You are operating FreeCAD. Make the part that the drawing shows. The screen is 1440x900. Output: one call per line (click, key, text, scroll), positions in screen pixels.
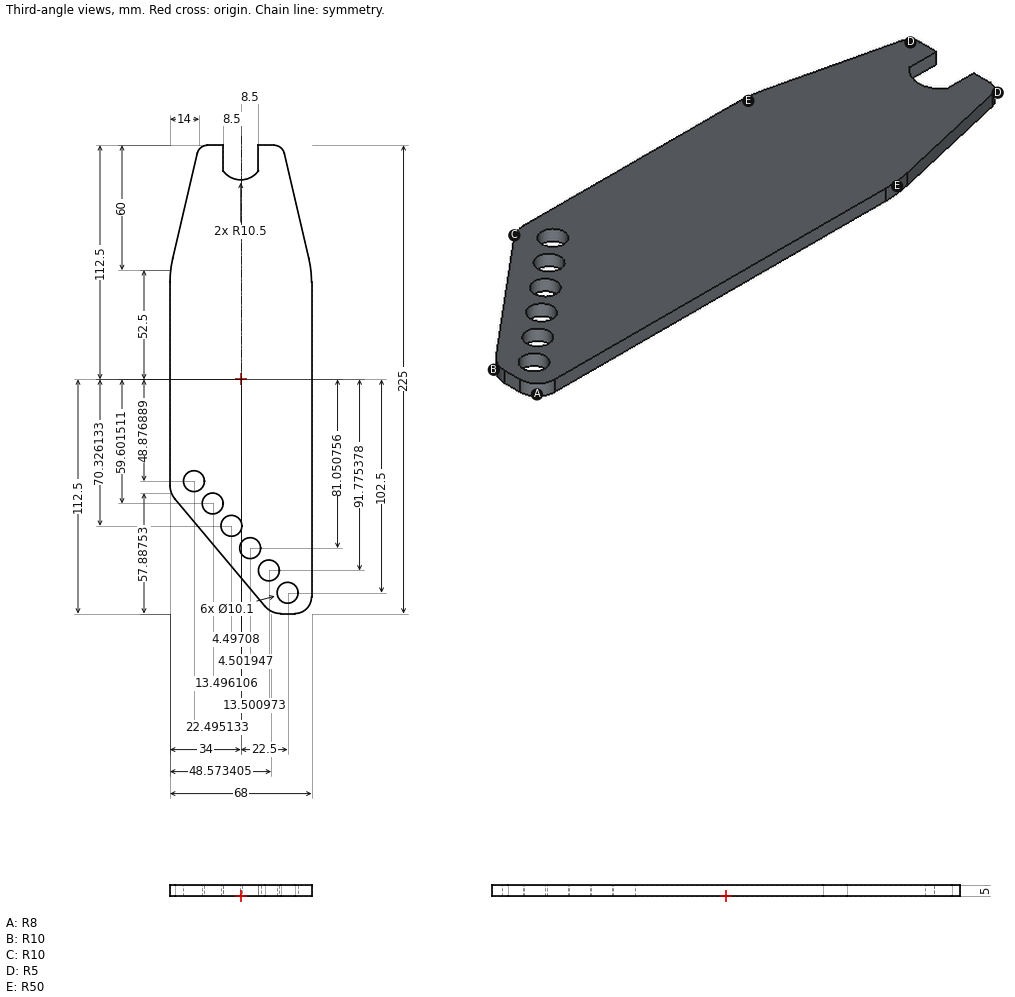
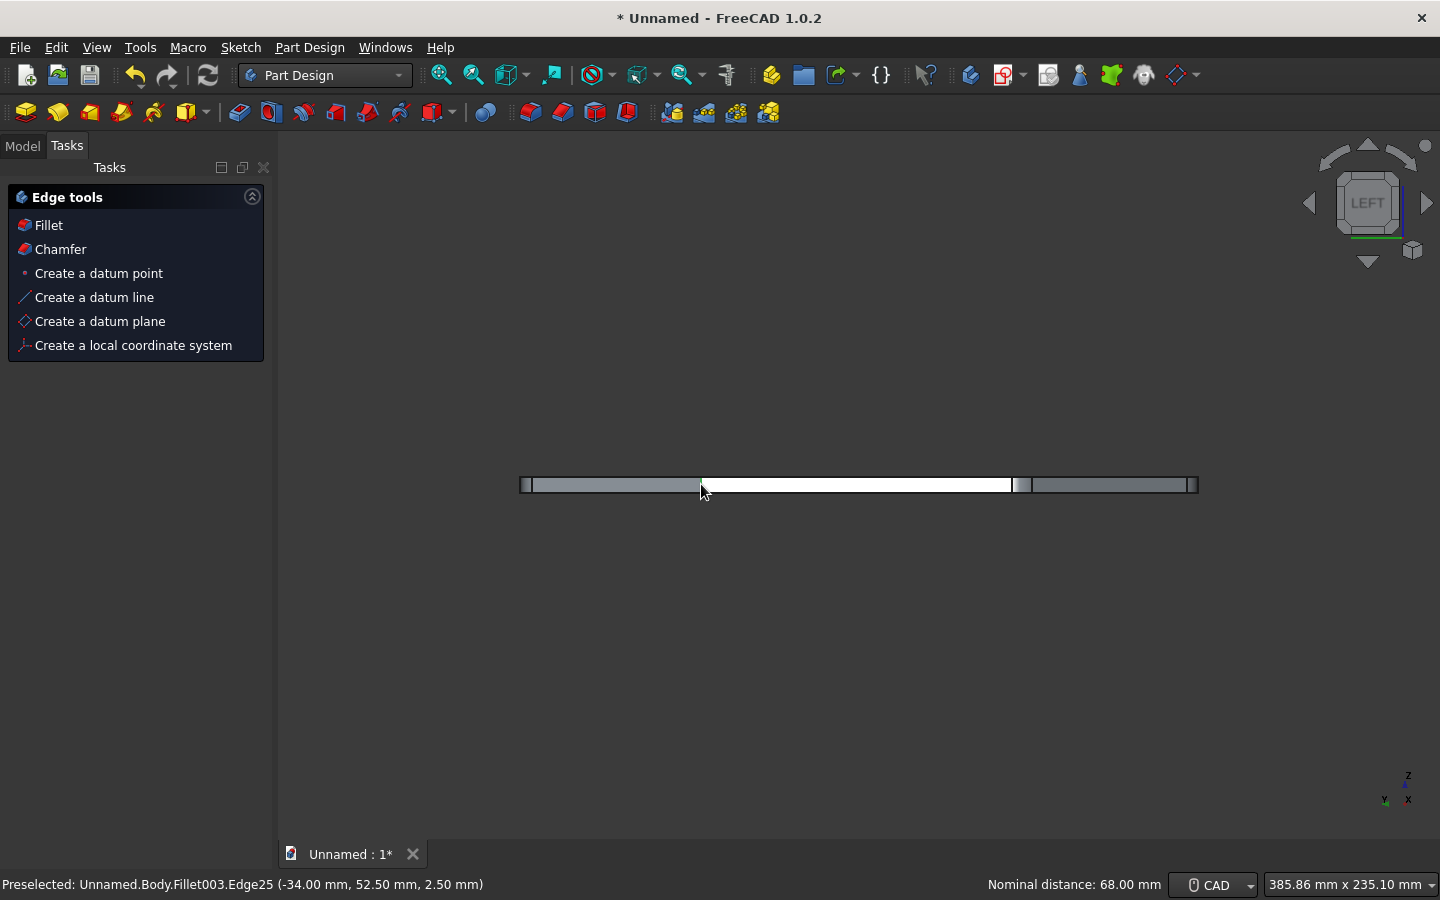
click(532, 112)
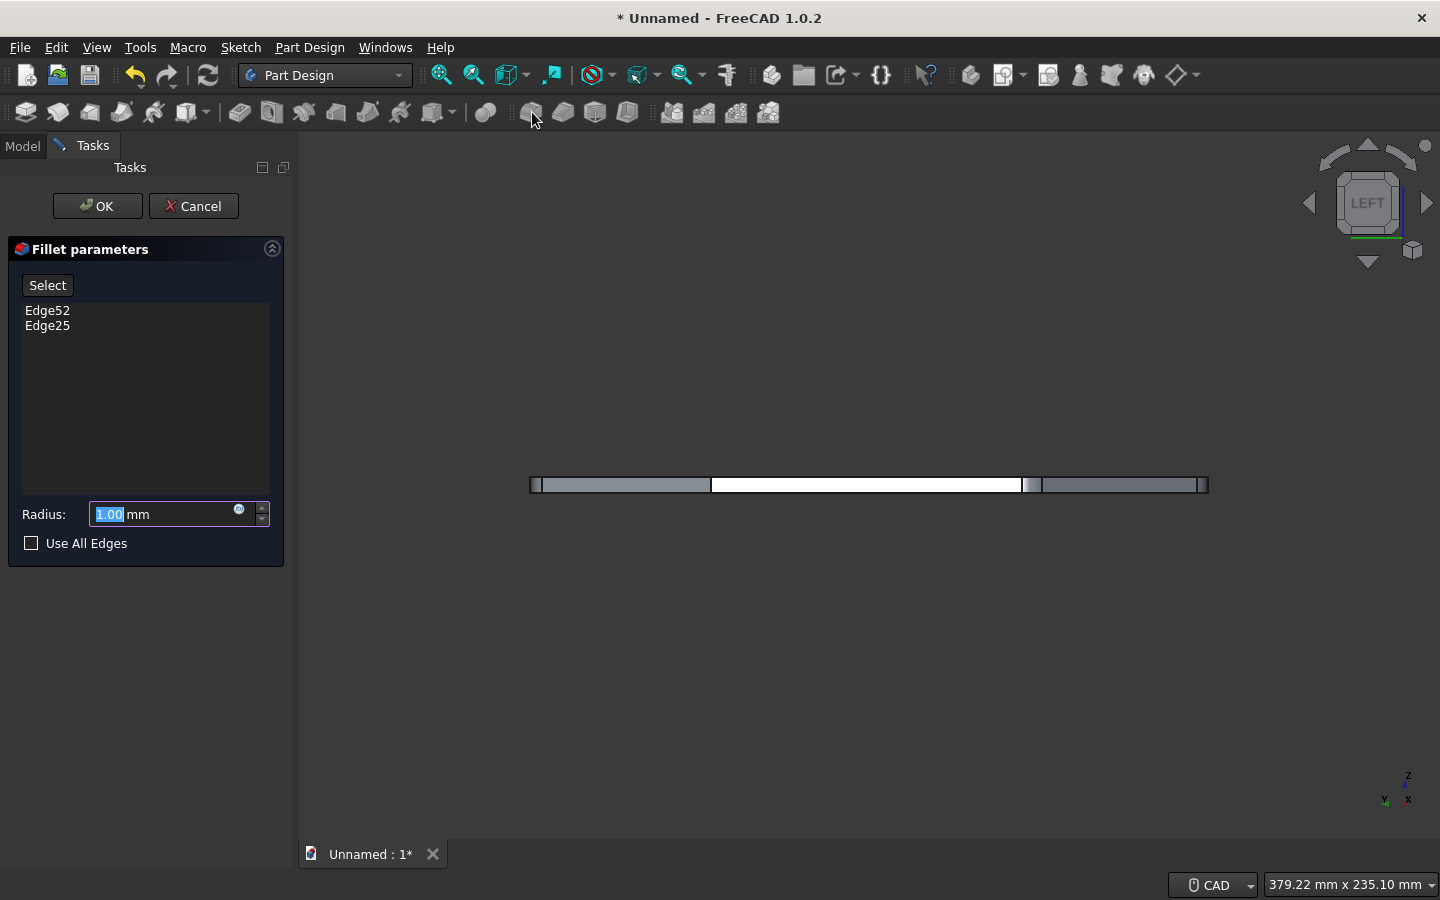
text(50)
key(Tab)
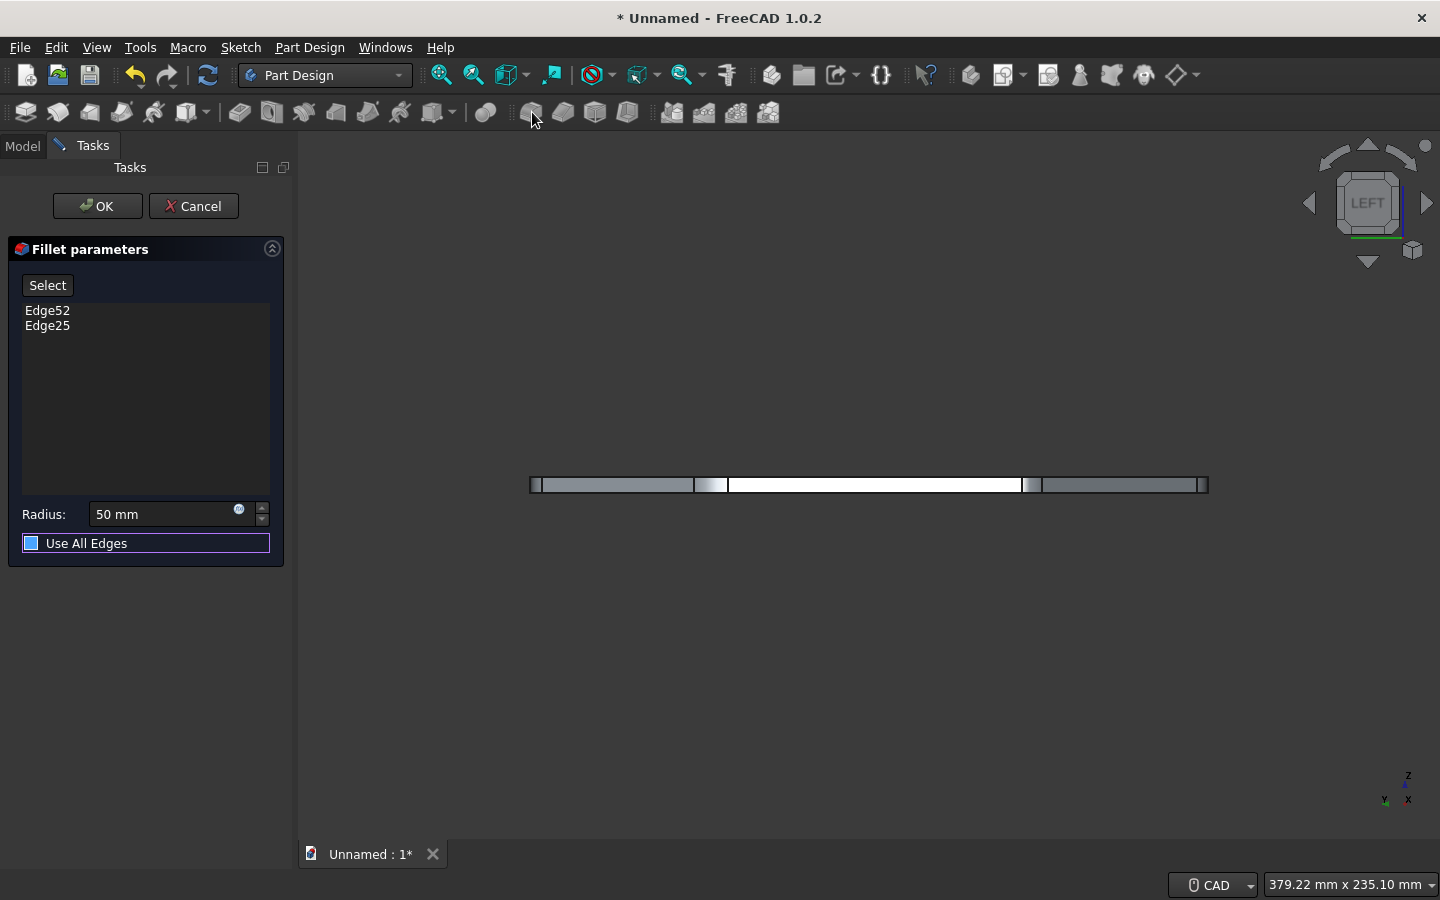
click(98, 206)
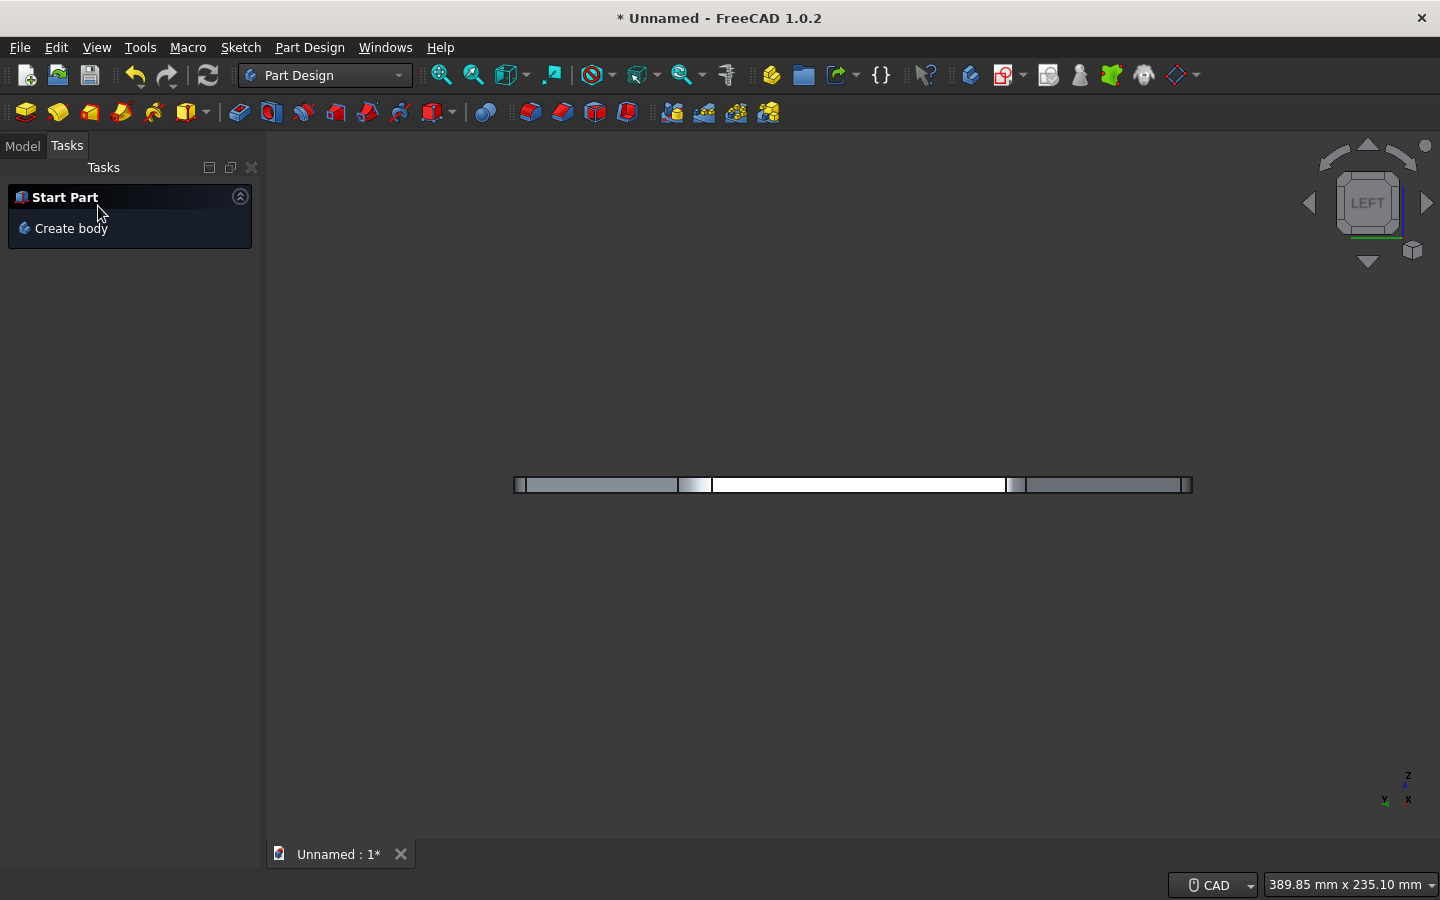
key(0)